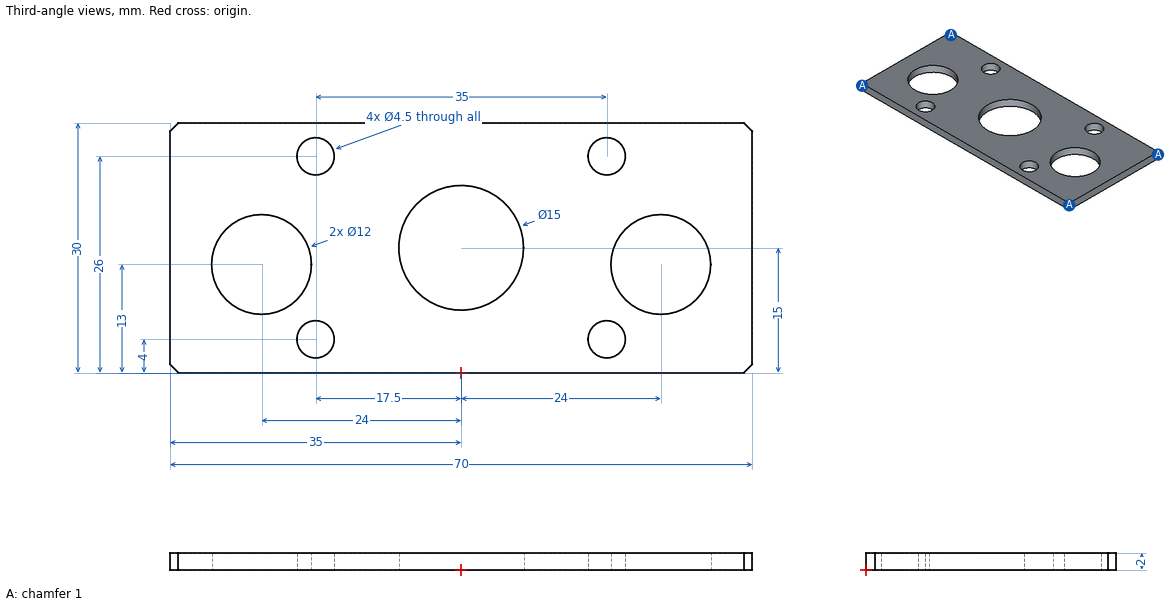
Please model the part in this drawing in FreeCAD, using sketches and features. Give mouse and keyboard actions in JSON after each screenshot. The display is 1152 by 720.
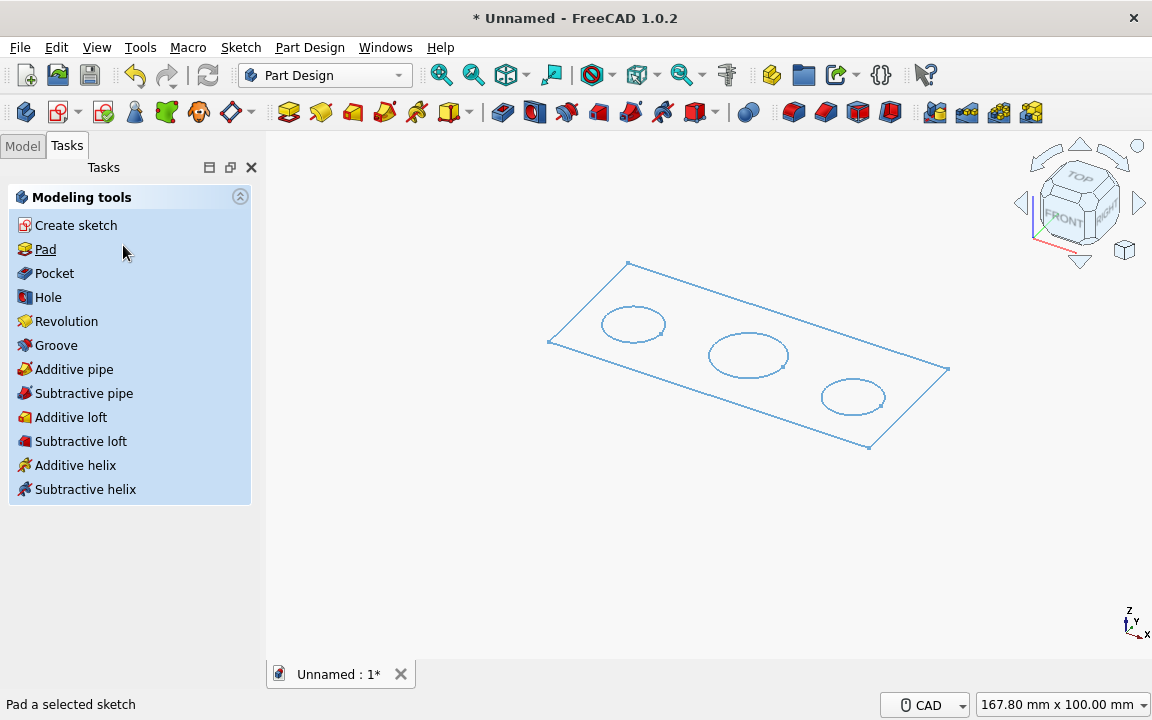
{"action": "left_click", "coordinate": [290, 112]}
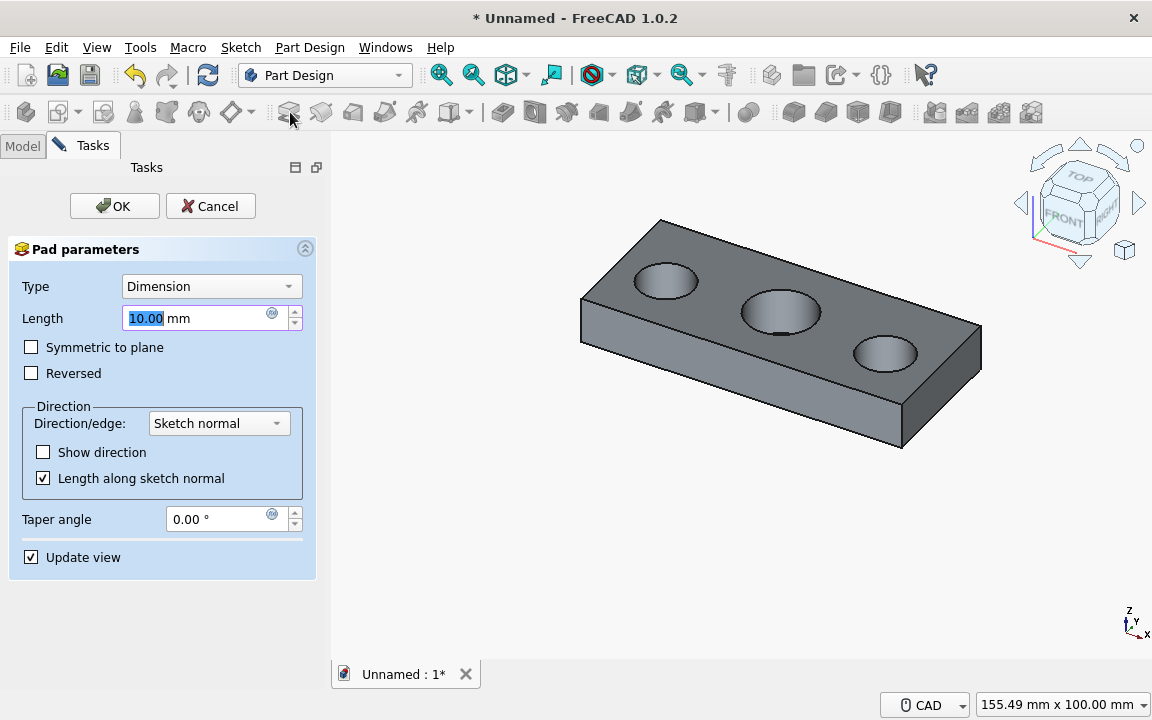
{"action": "type", "text": "2"}
{"action": "key", "text": "Tab"}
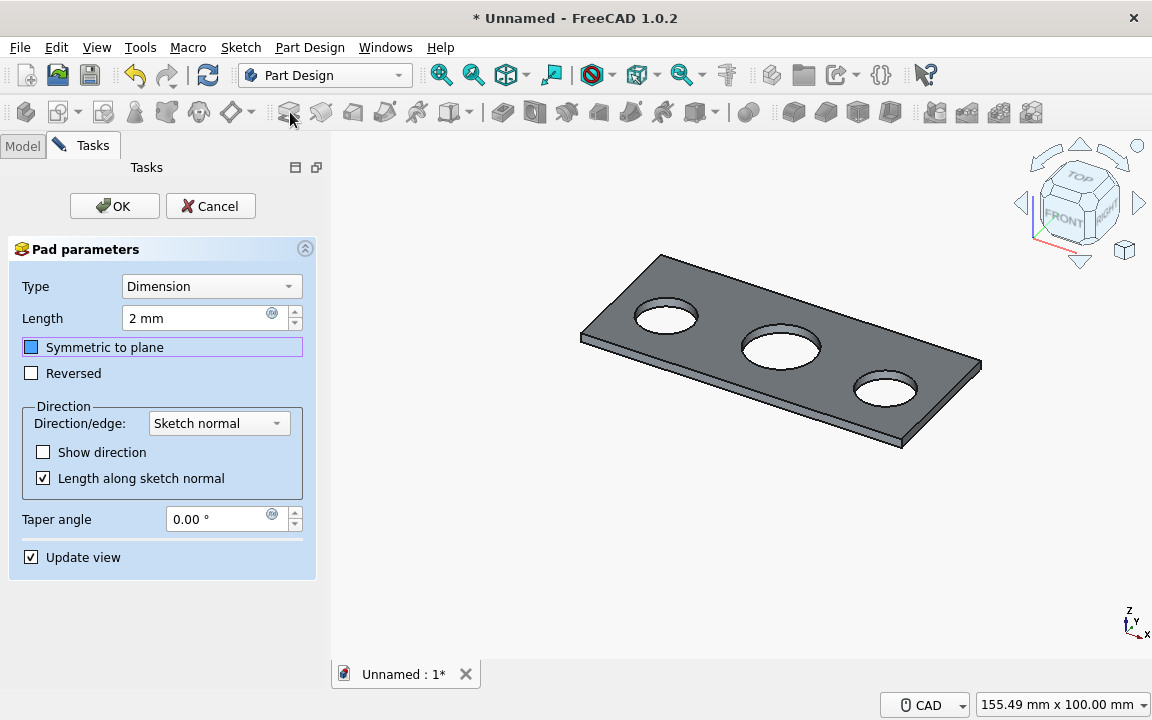
{"action": "left_click", "coordinate": [115, 206]}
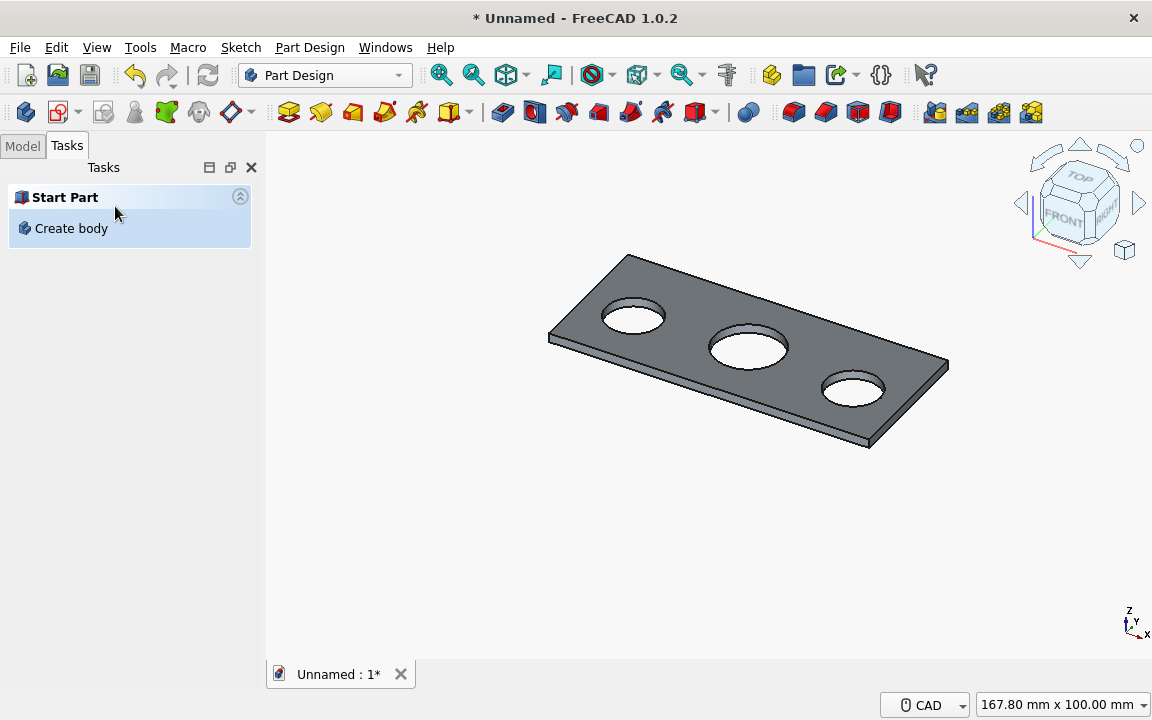
{"action": "left_click", "coordinate": [680, 353]}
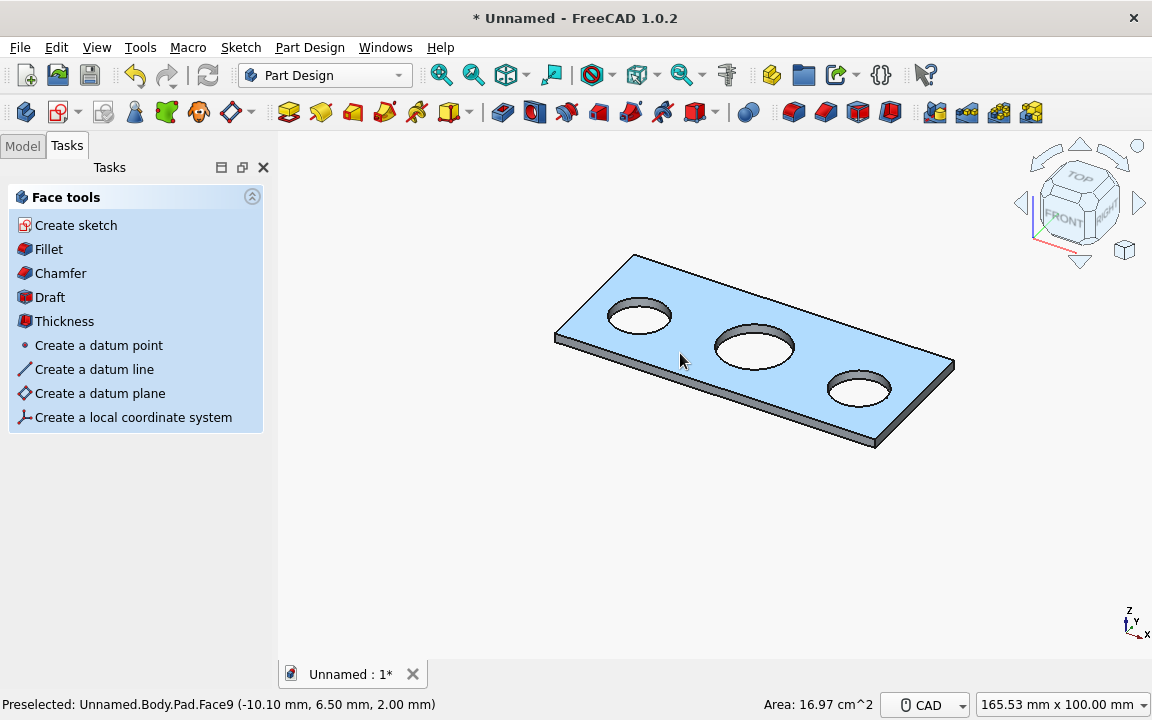
{"action": "left_click", "coordinate": [58, 112]}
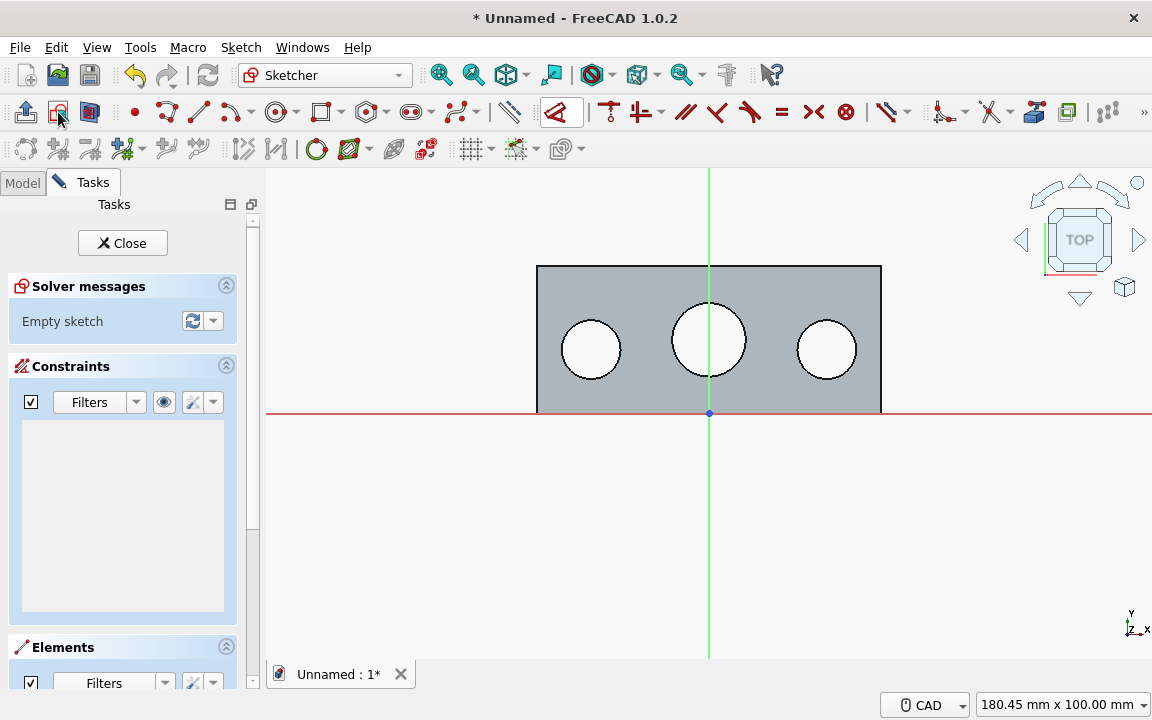
{"action": "scroll", "coordinate": [765, 288], "scroll_direction": "up", "scroll_amount": 4}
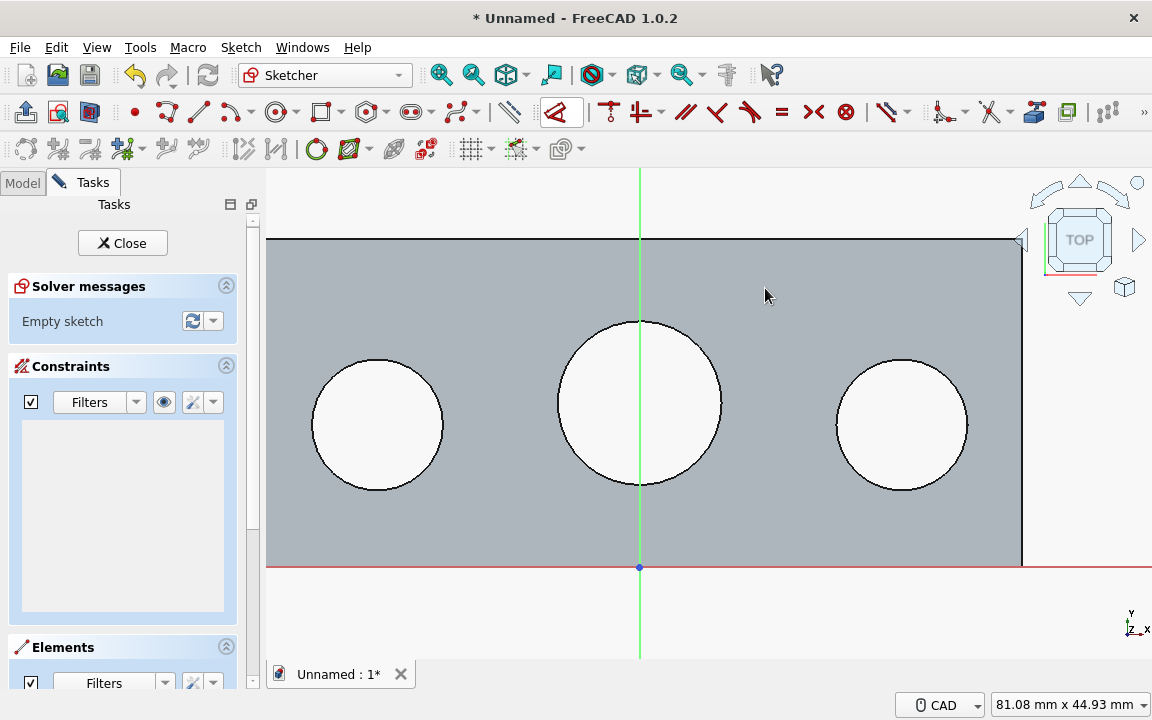
{"action": "left_click", "coordinate": [276, 112]}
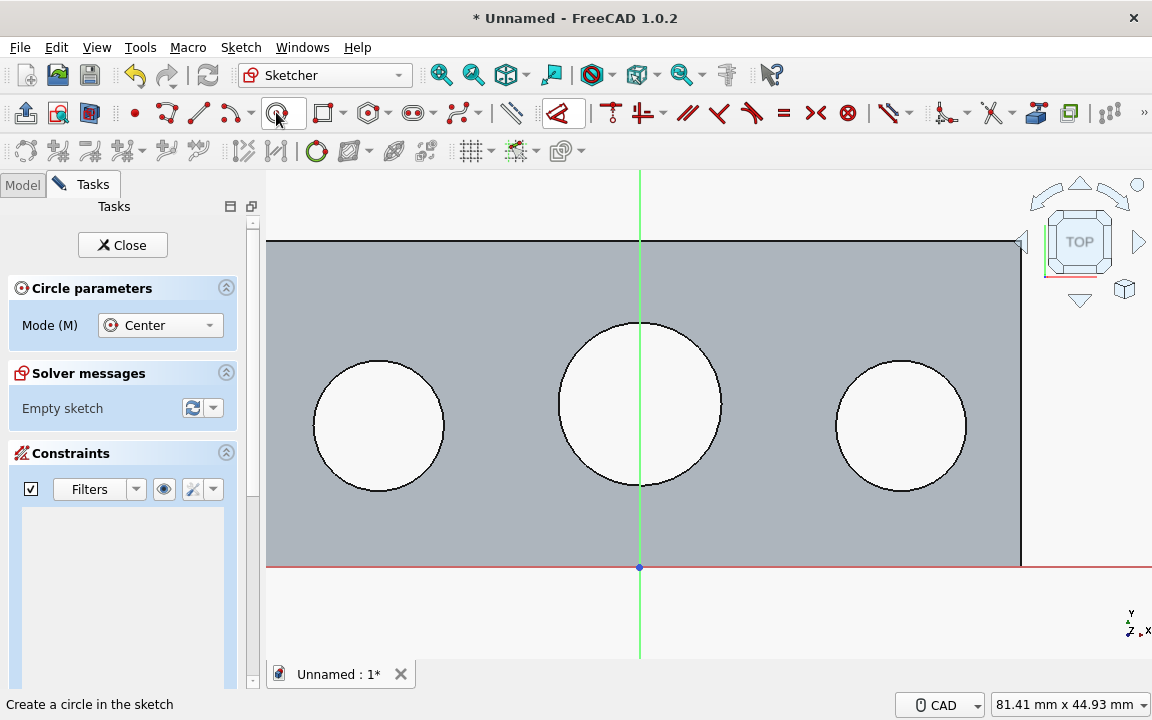
{"action": "left_click", "coordinate": [450, 284]}
{"action": "left_click", "coordinate": [467, 267]}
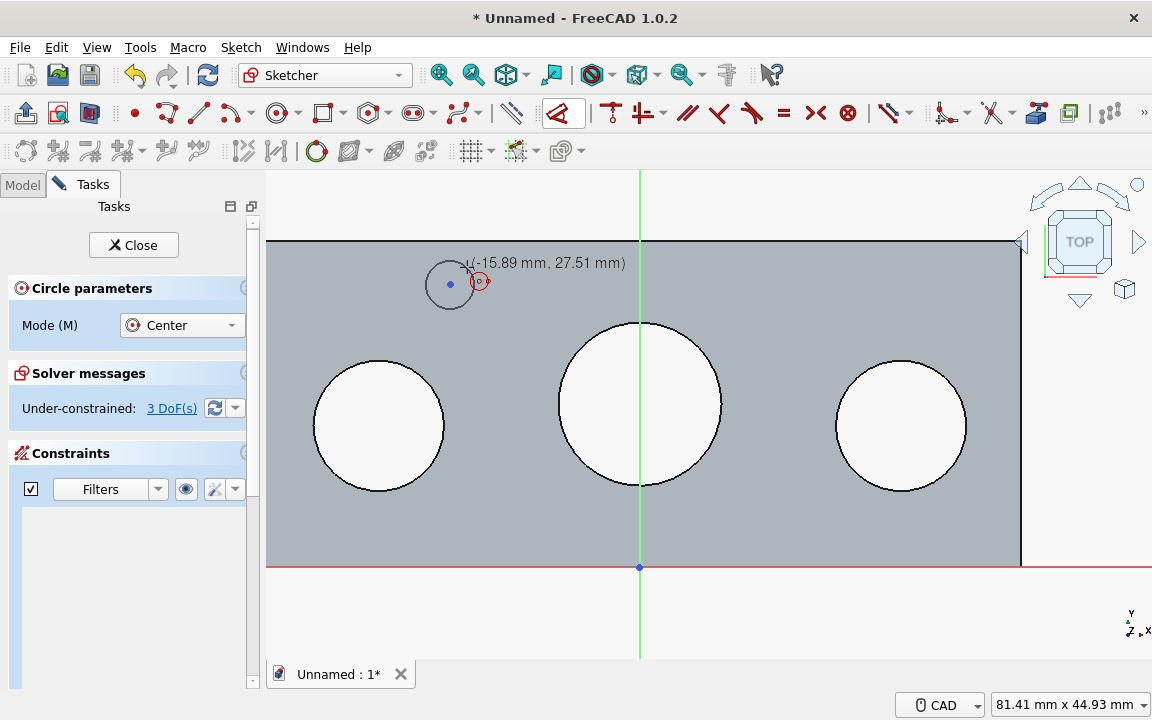
{"action": "left_click", "coordinate": [830, 284]}
{"action": "left_click", "coordinate": [848, 267]}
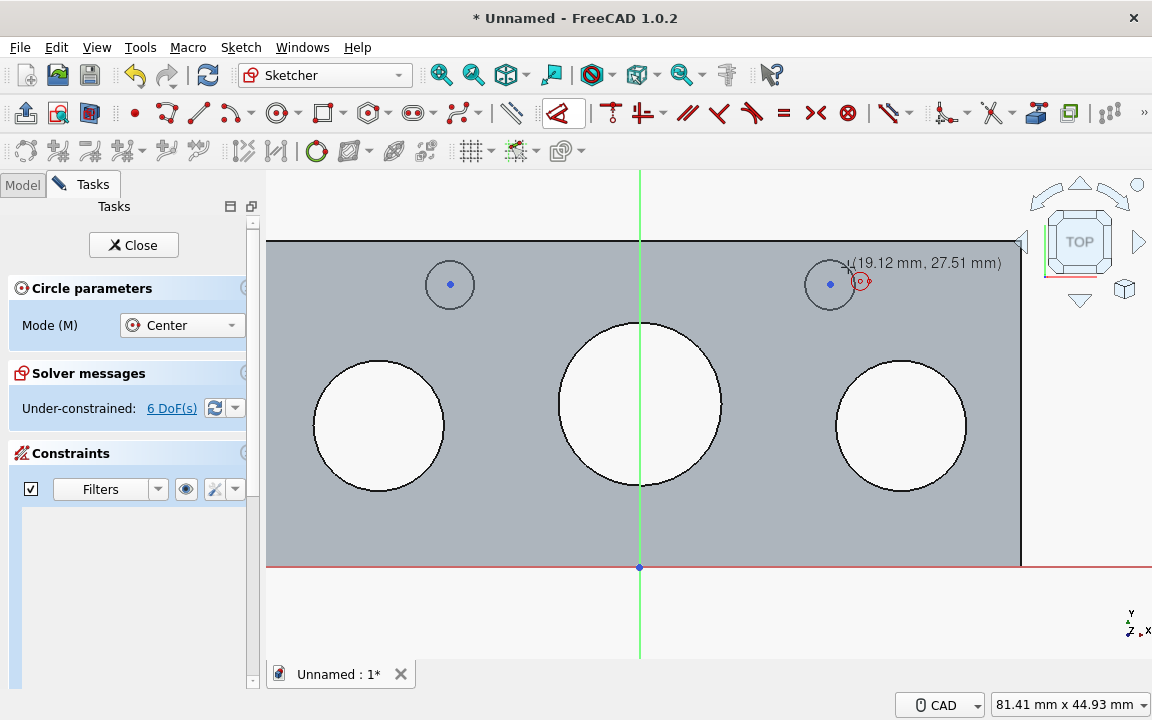
{"action": "left_click", "coordinate": [450, 524]}
{"action": "left_click", "coordinate": [467, 507]}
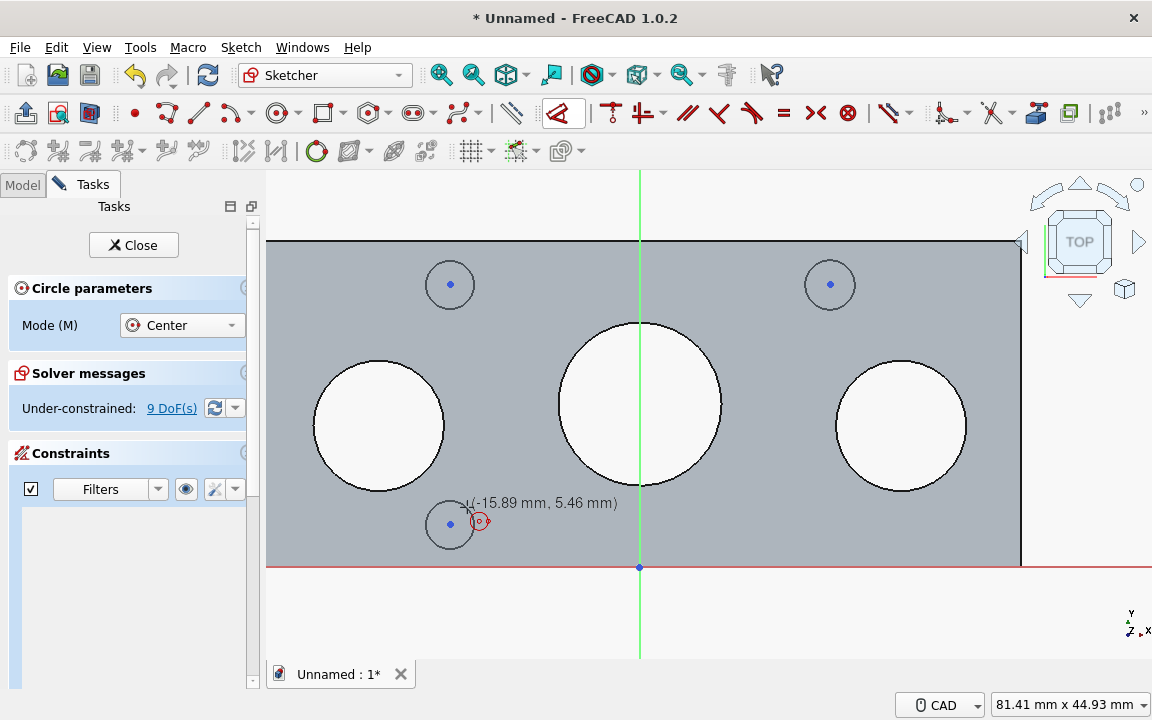
{"action": "left_click", "coordinate": [830, 524]}
{"action": "left_click", "coordinate": [848, 507]}
{"action": "key", "text": "Escape"}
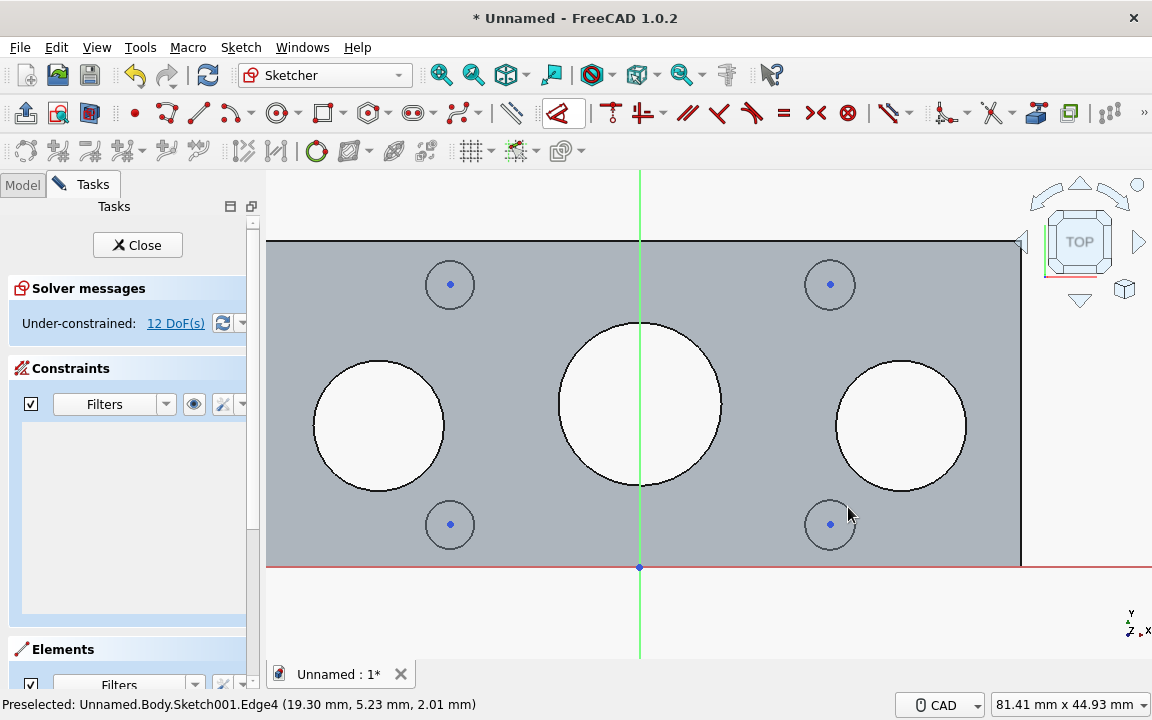
{"action": "left_click", "coordinate": [467, 268]}